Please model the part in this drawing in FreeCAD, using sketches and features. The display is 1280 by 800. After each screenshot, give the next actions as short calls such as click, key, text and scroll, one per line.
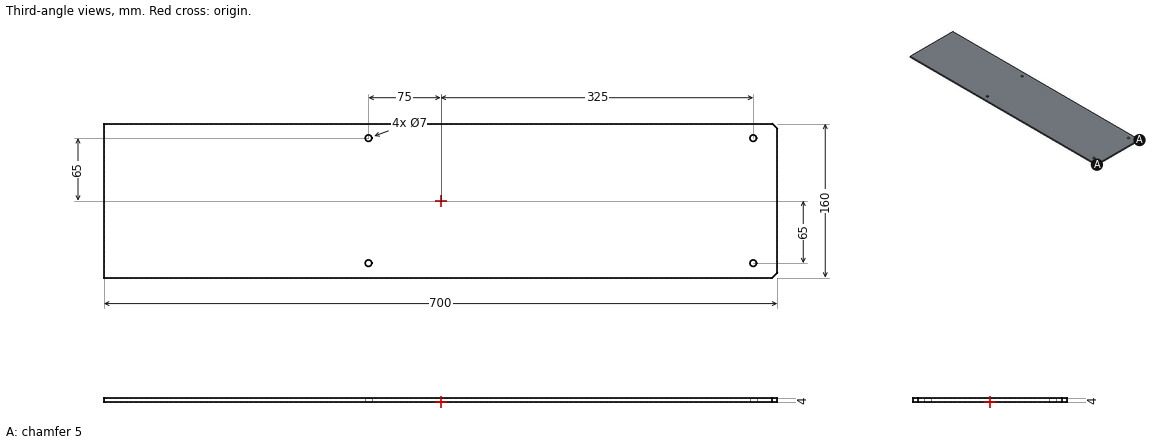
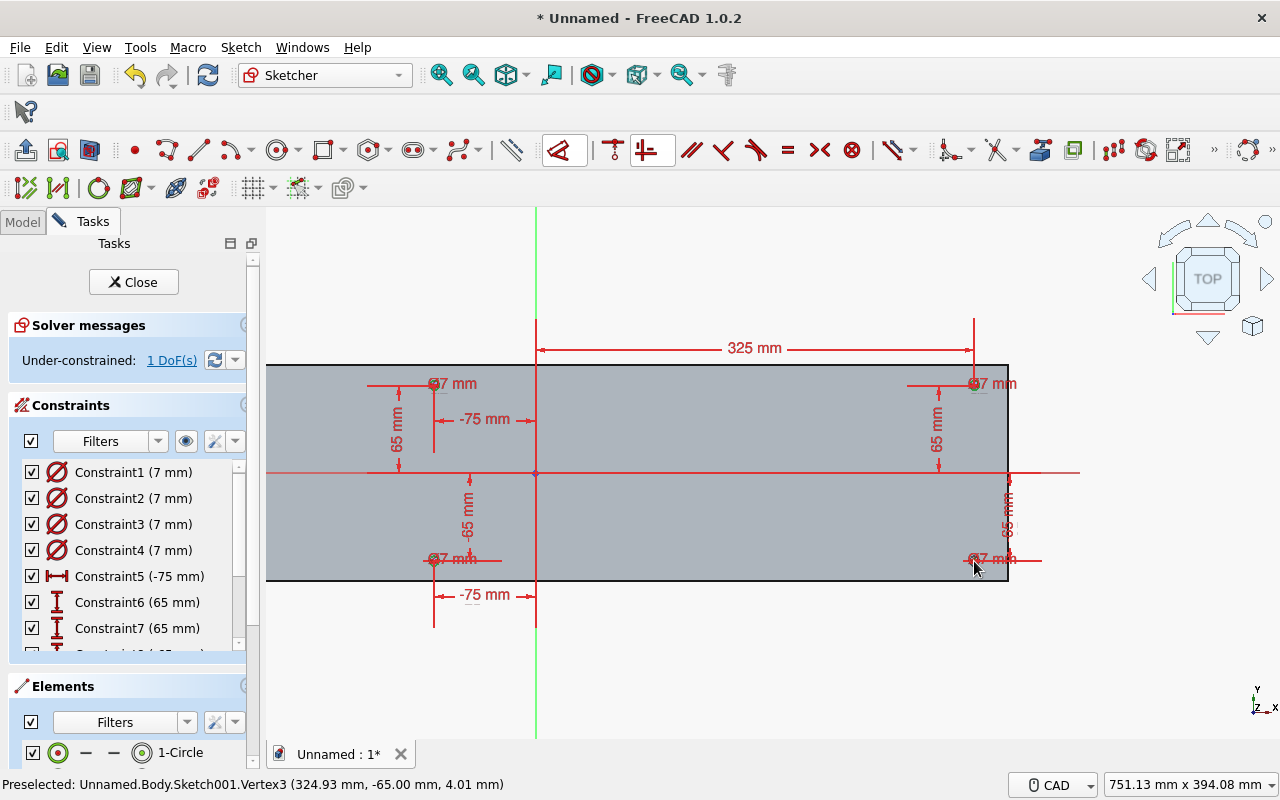
key(l)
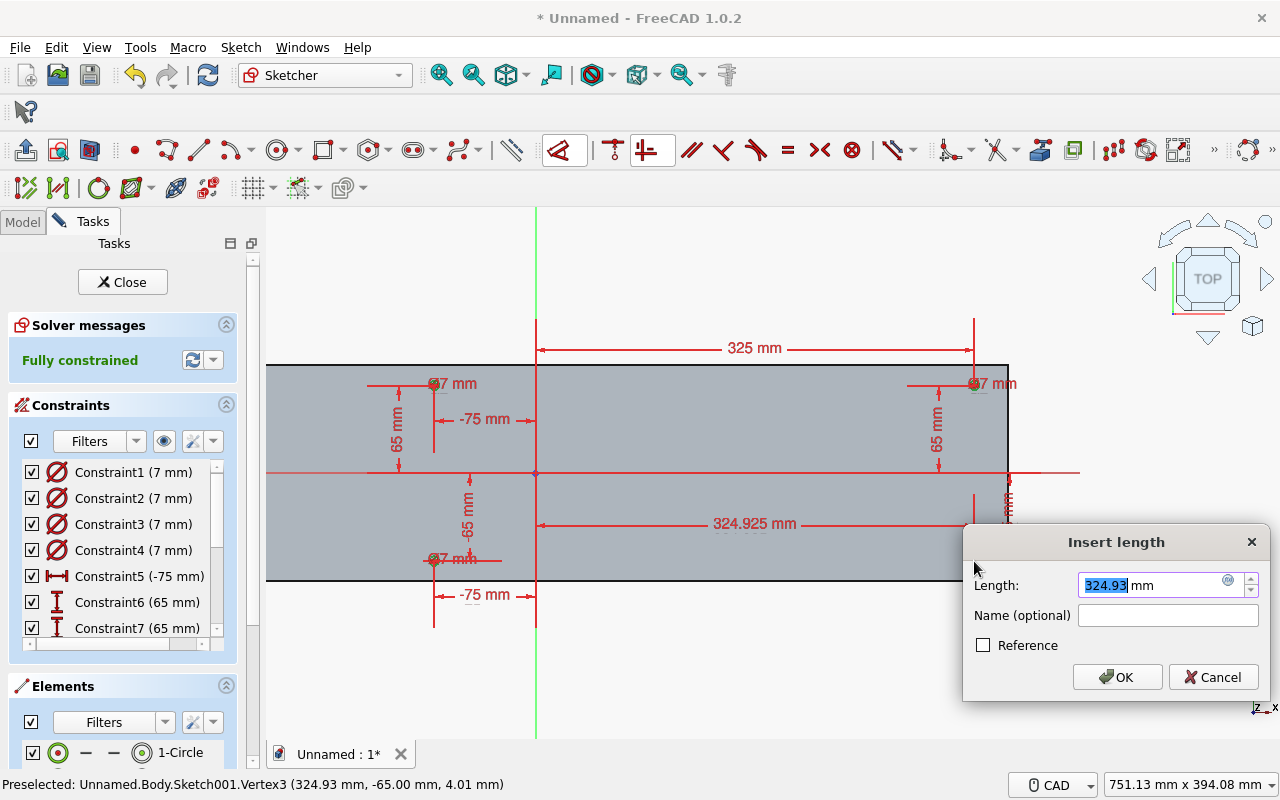
text(325)
key(Return)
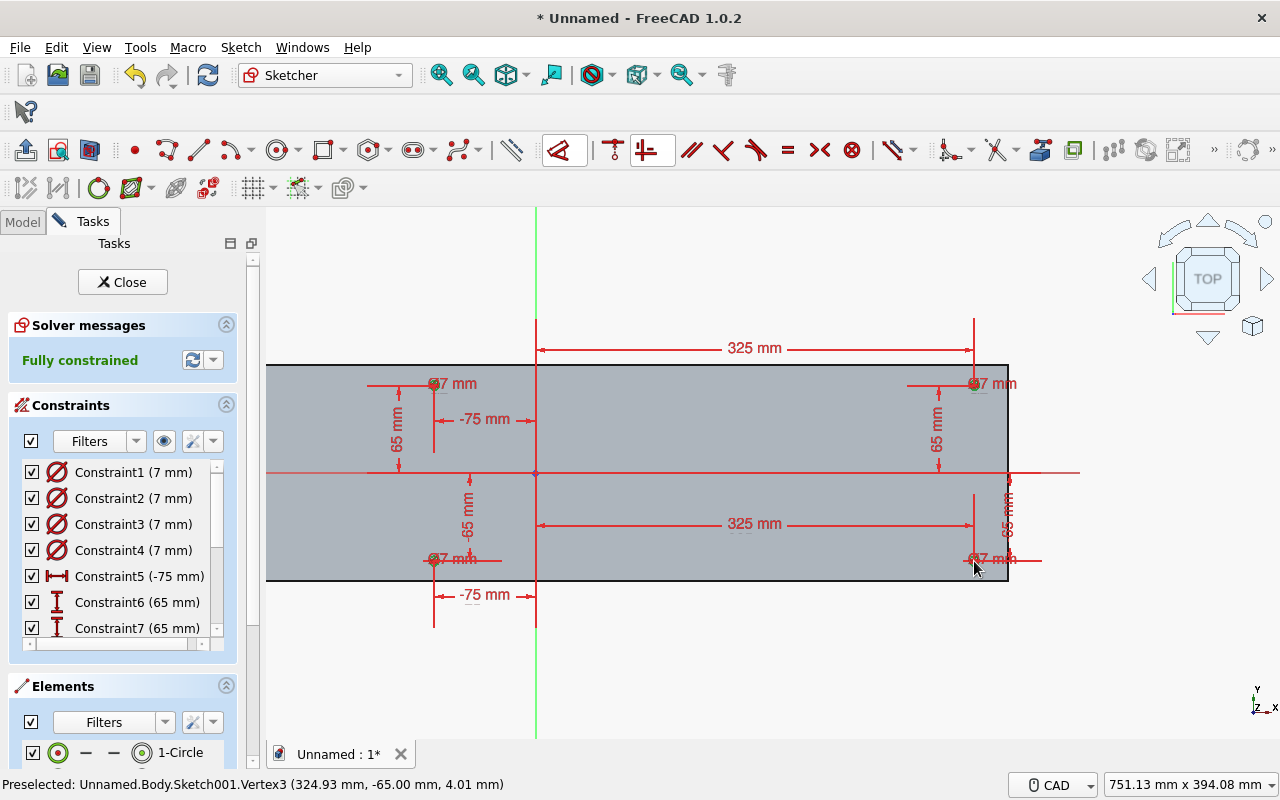
click(123, 282)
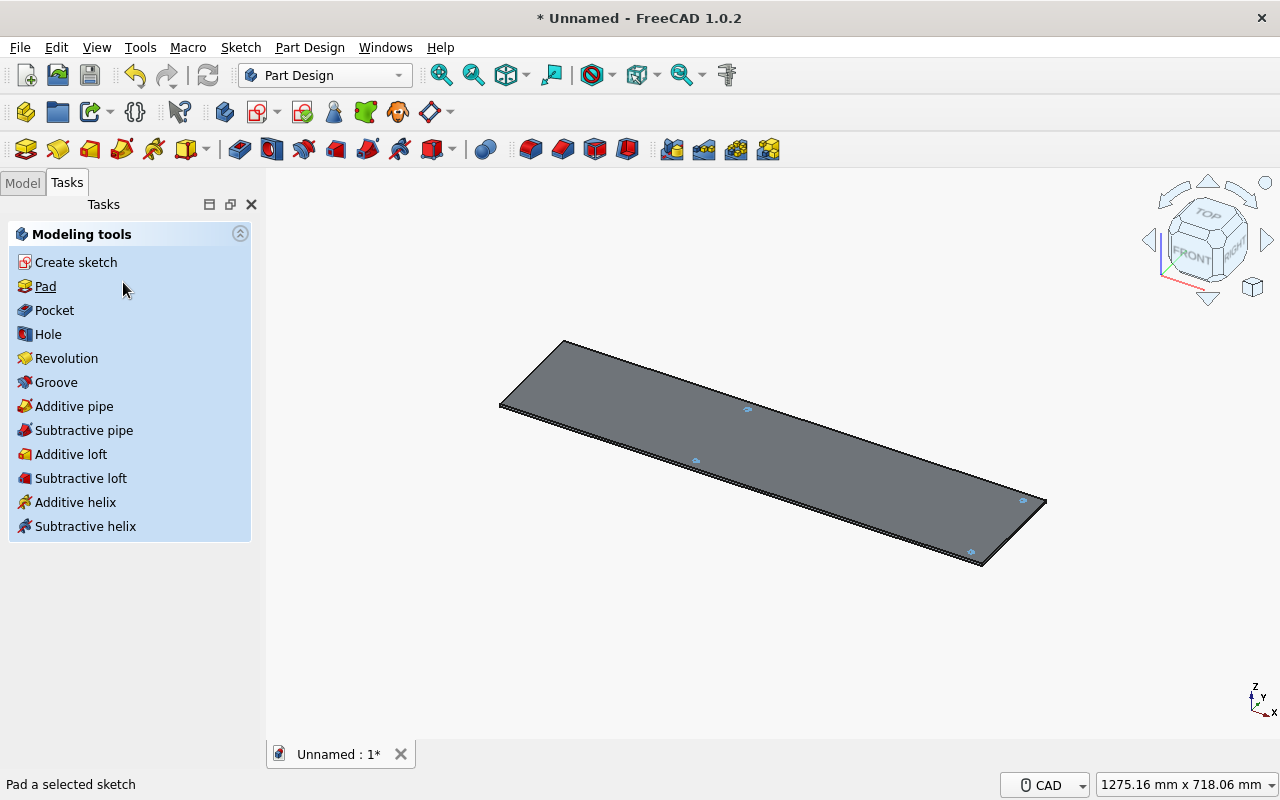
click(240, 150)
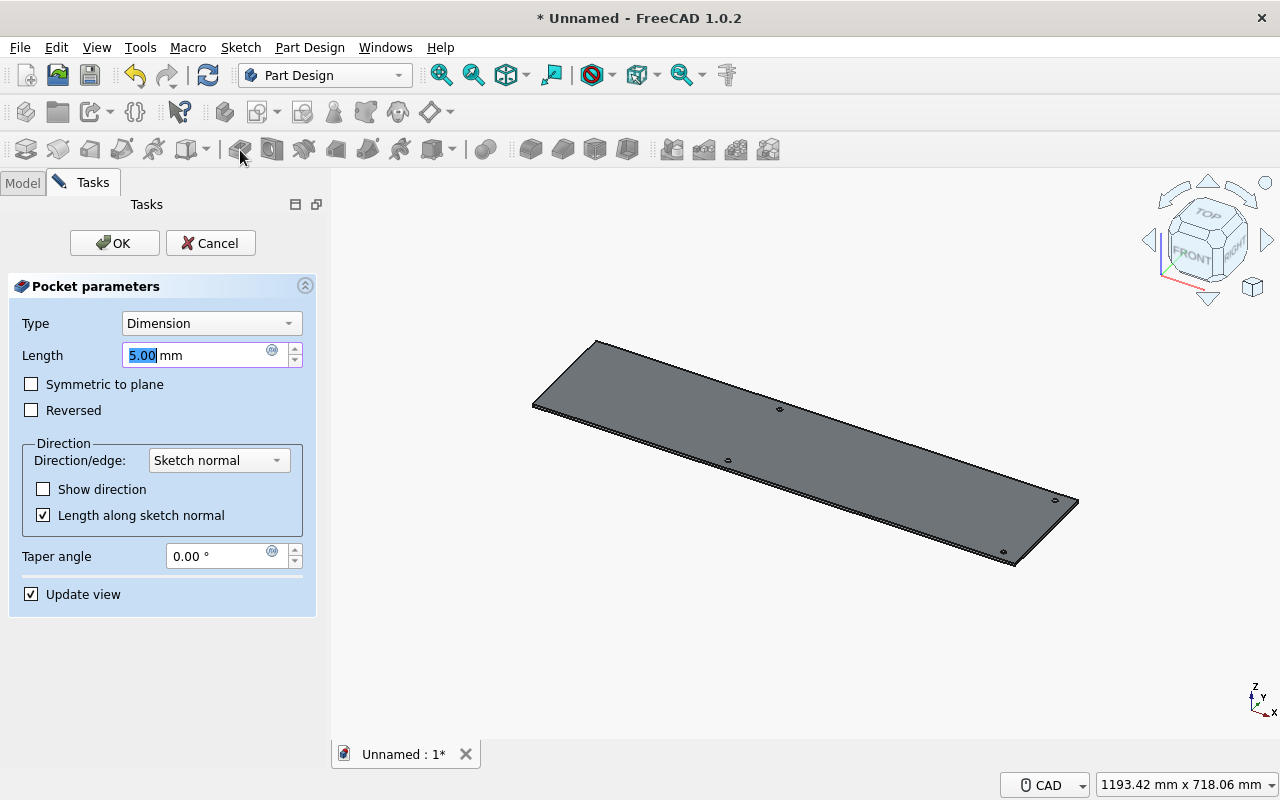
text(4)
key(Tab)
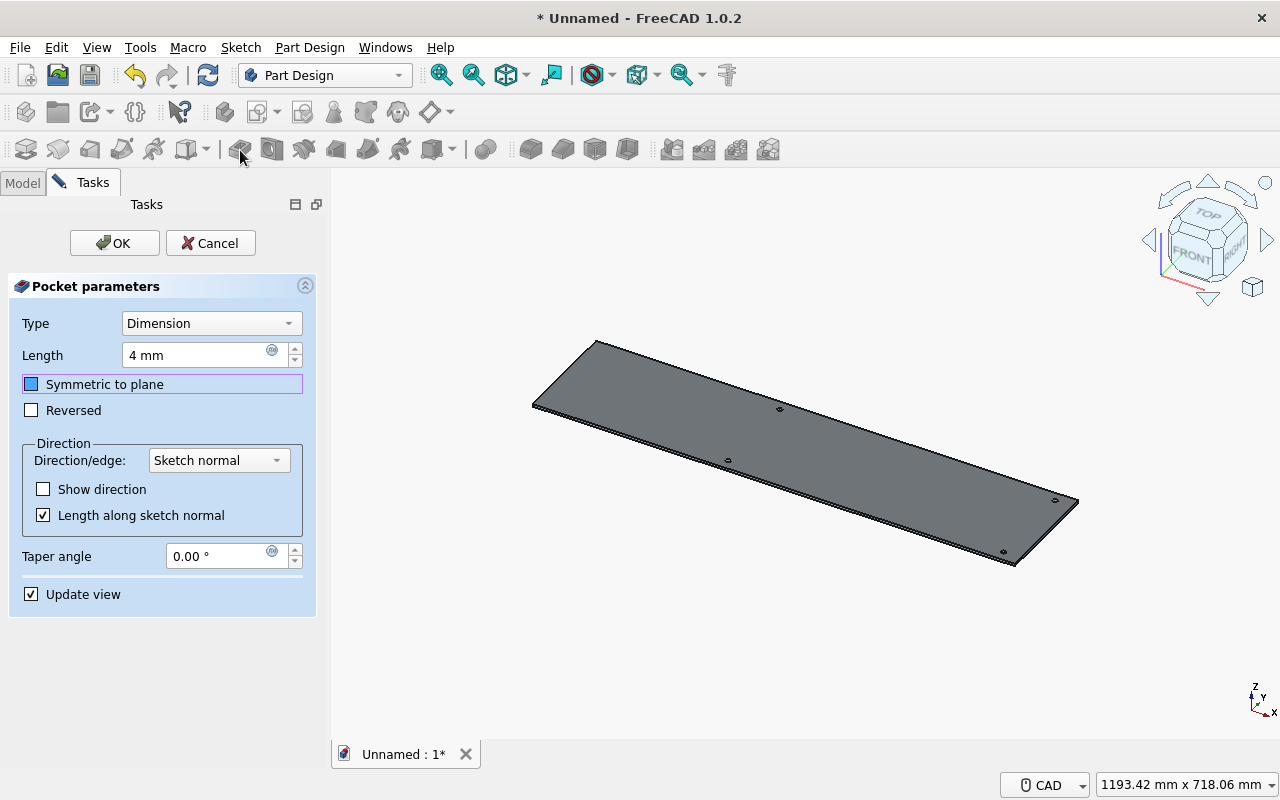
click(115, 243)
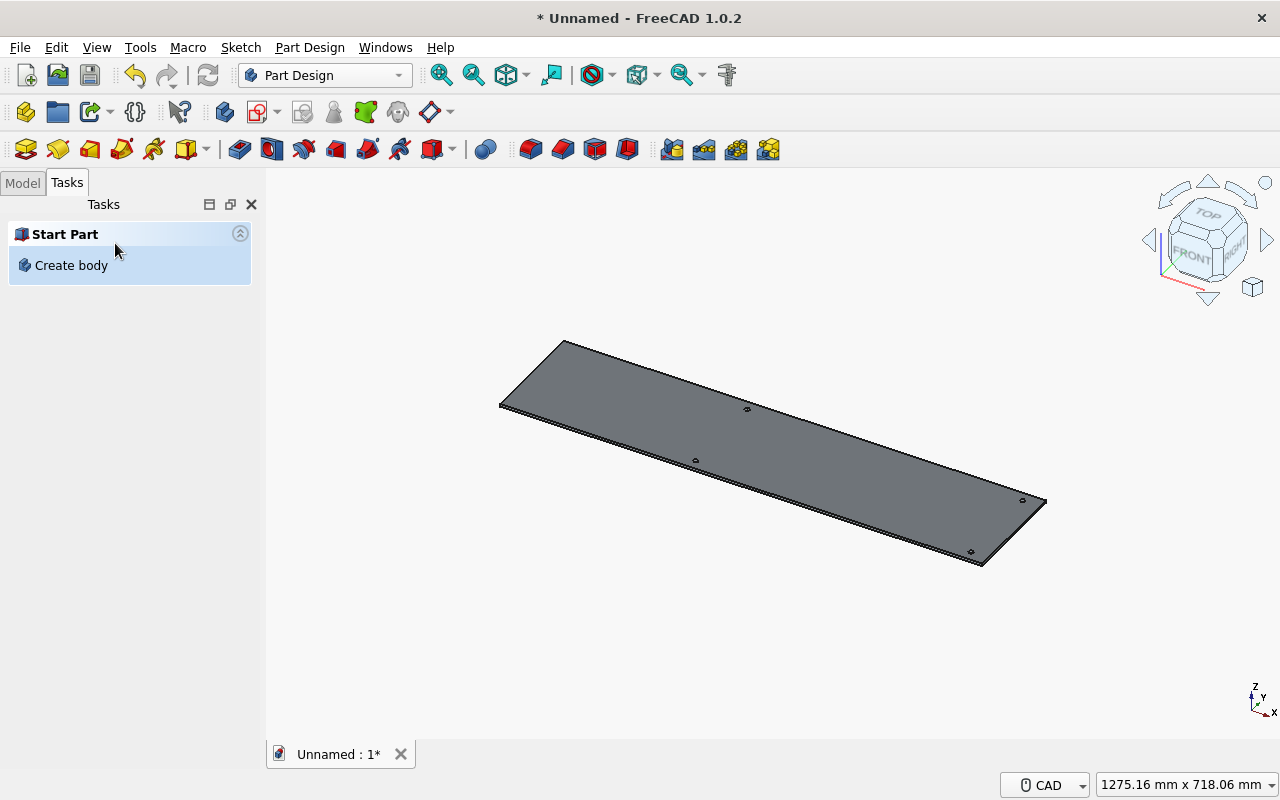
scroll(1046, 501, up, 13)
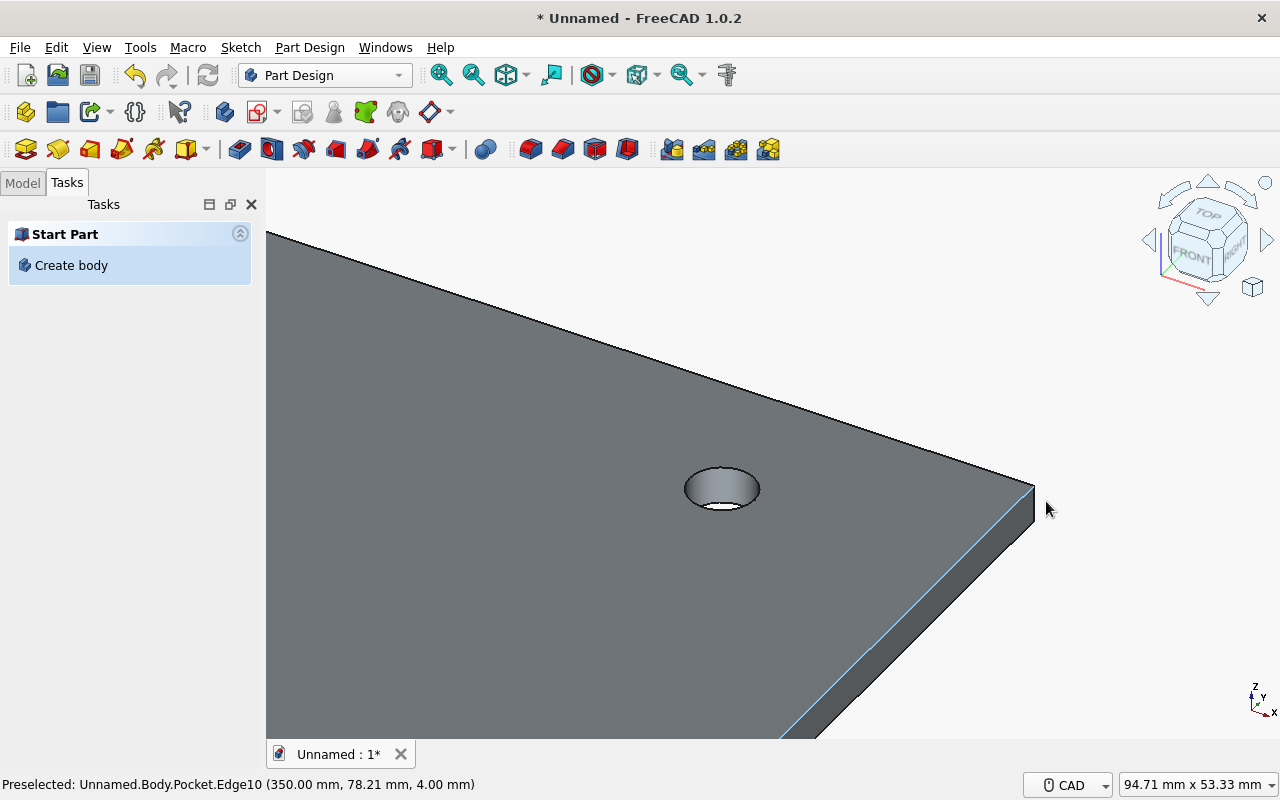
click(442, 76)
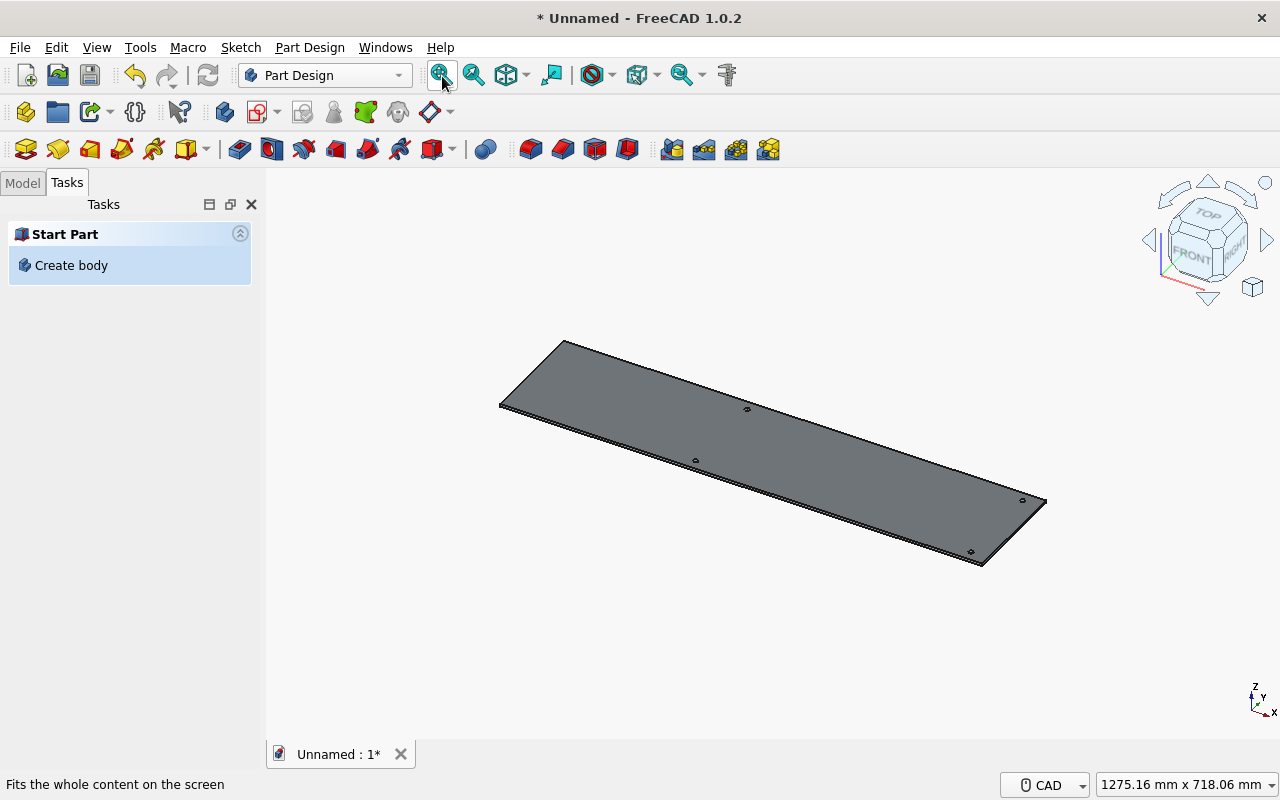
key(0)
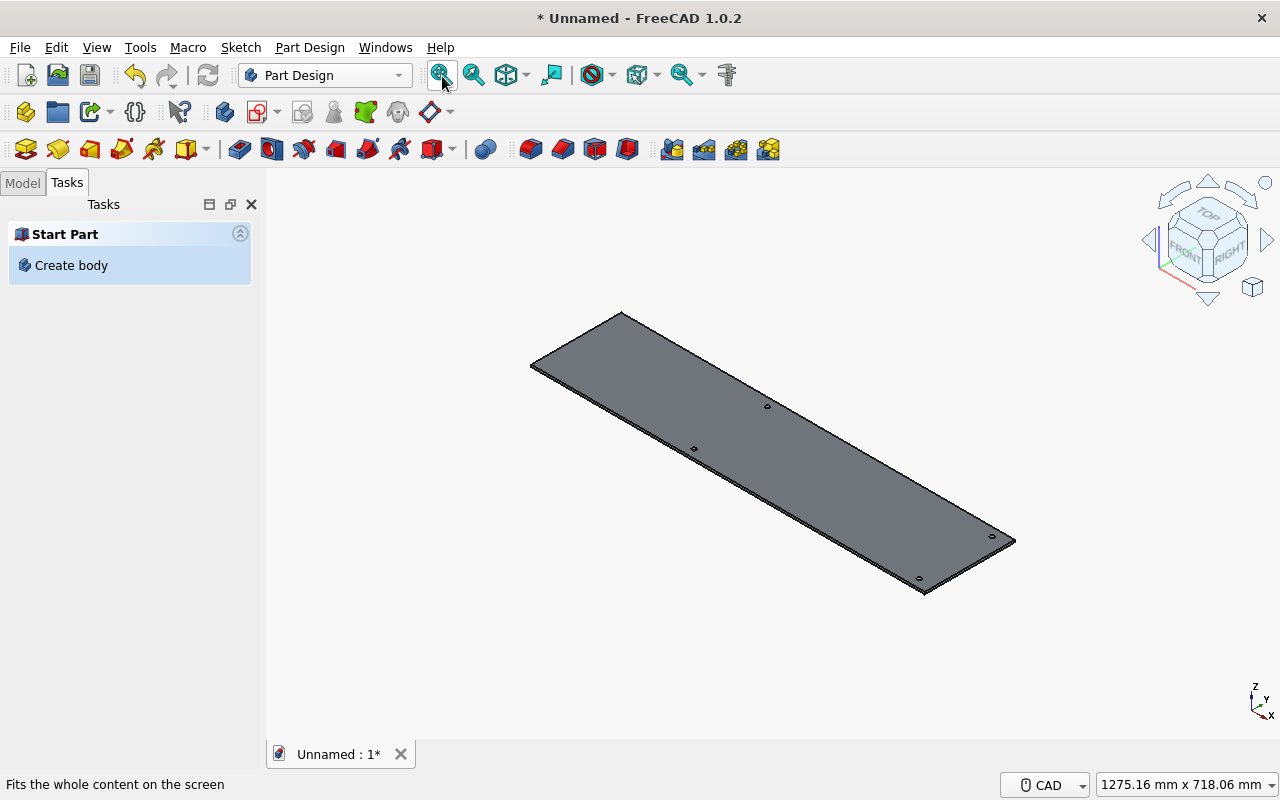
scroll(1015, 540, up, 13)